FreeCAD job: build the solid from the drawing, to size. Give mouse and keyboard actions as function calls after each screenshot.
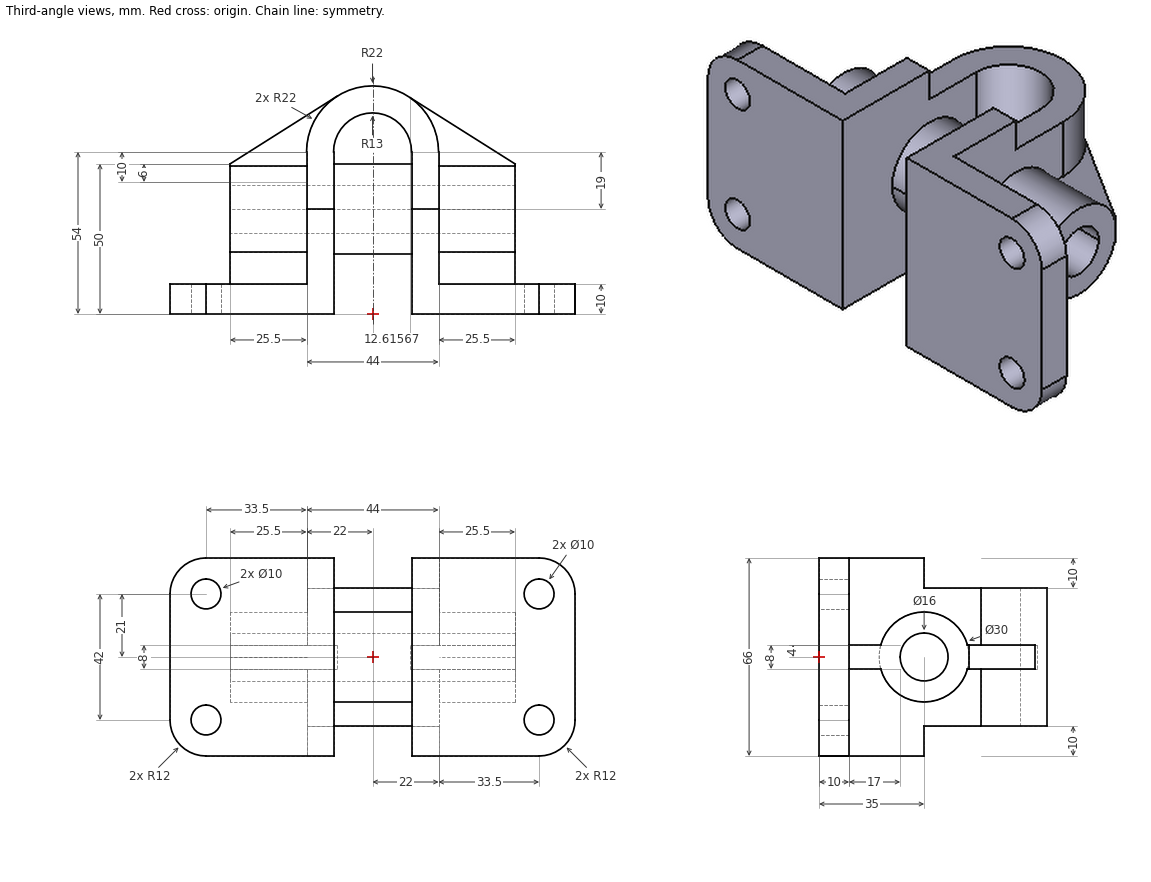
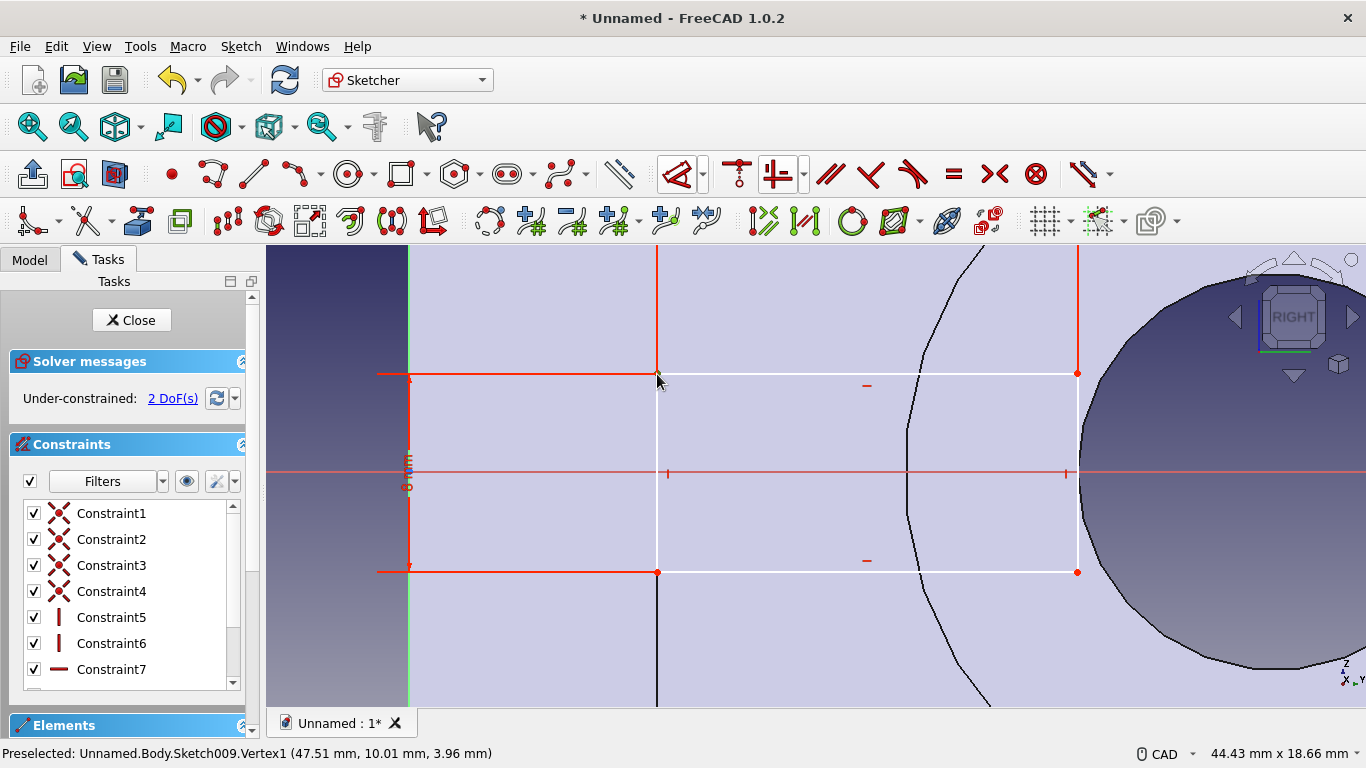
click(702, 174)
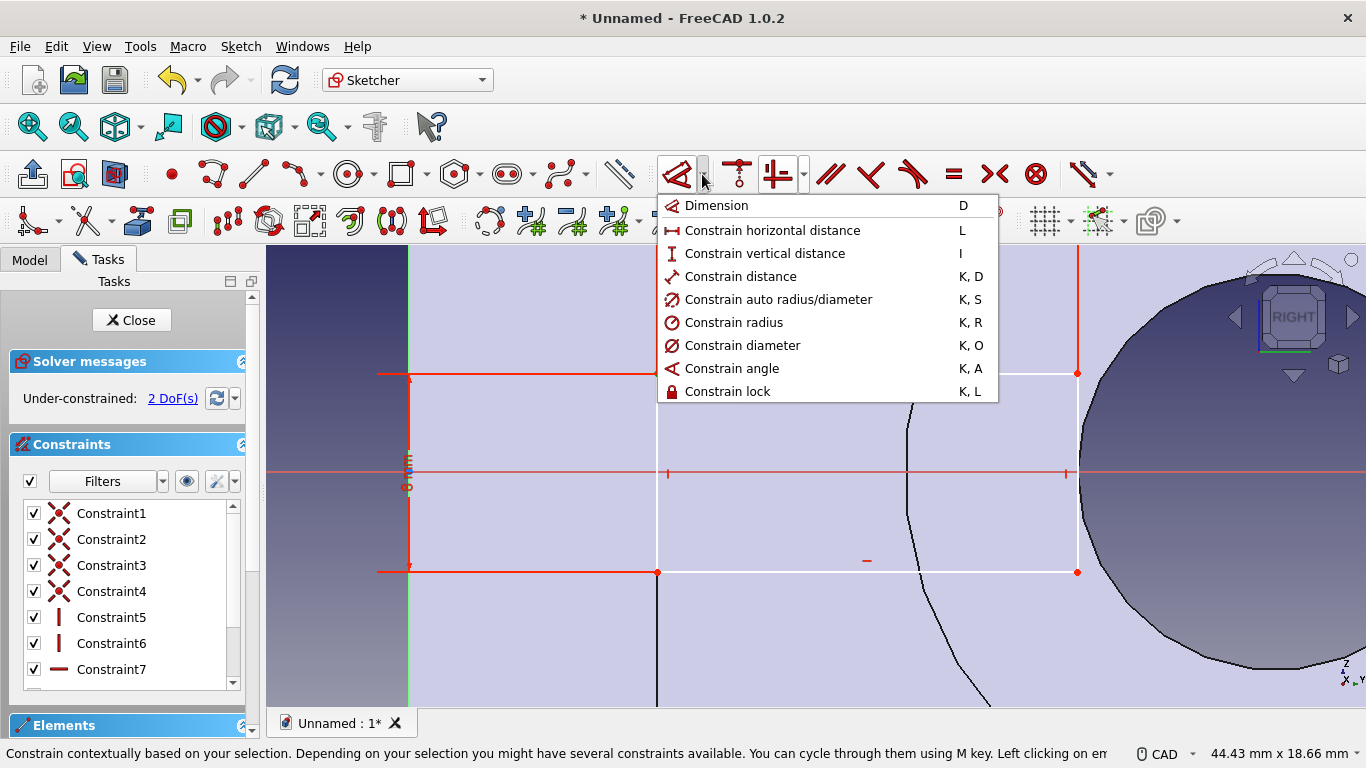
click(828, 254)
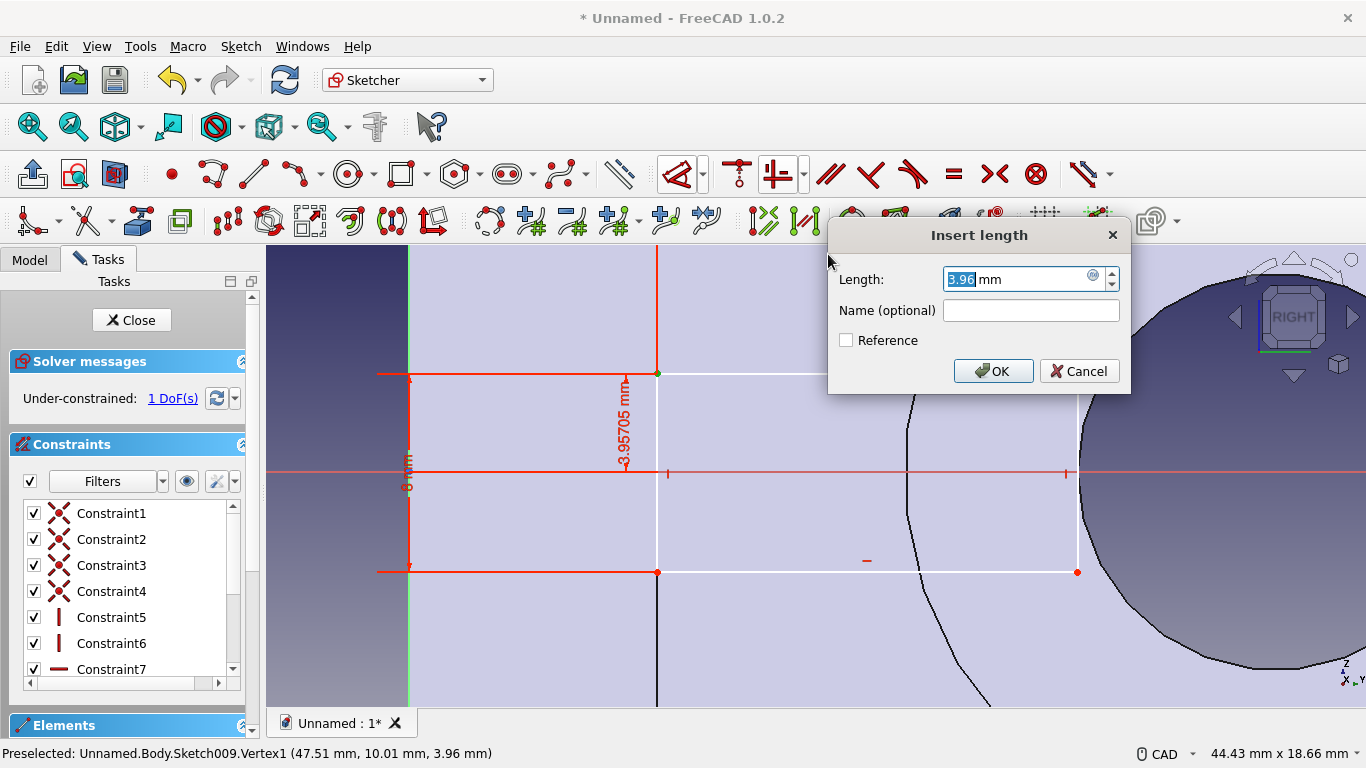
text(4)
key(Return)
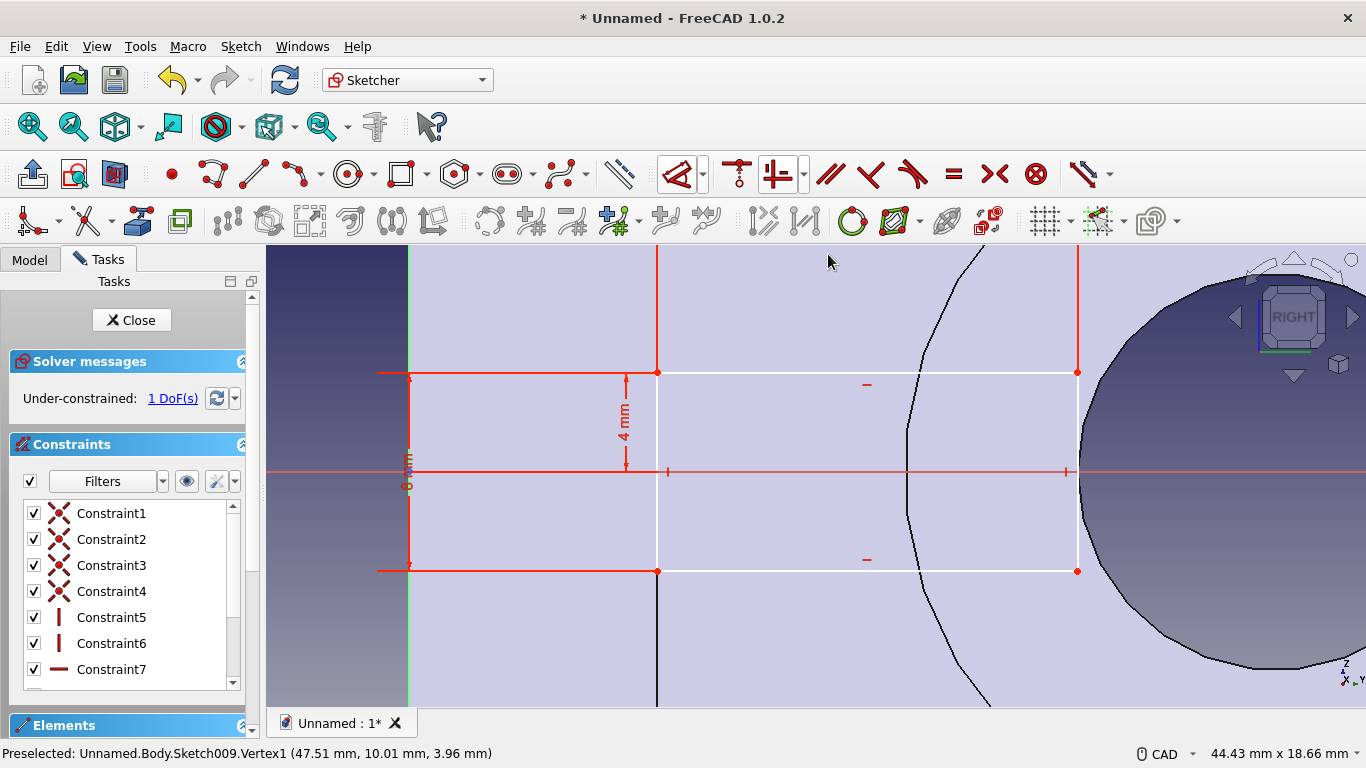
click(657, 373)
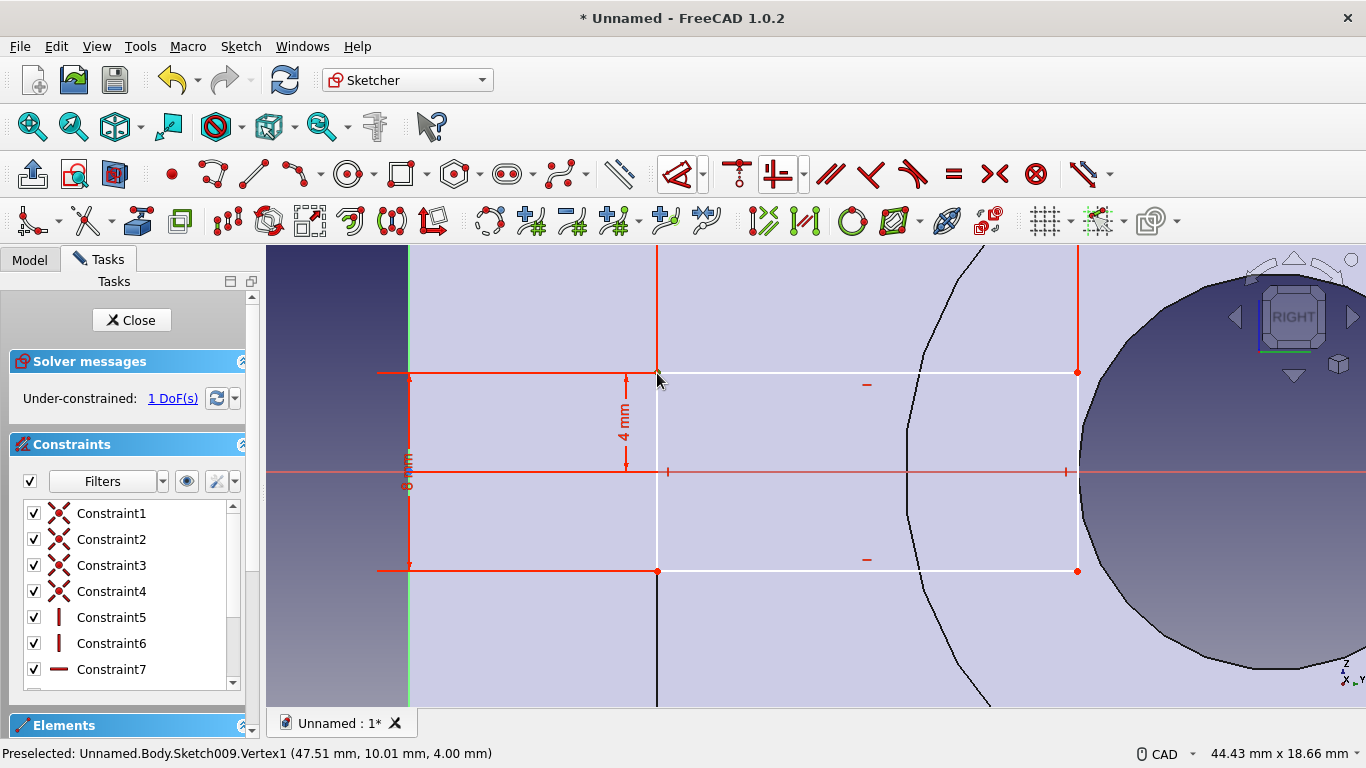
click(702, 174)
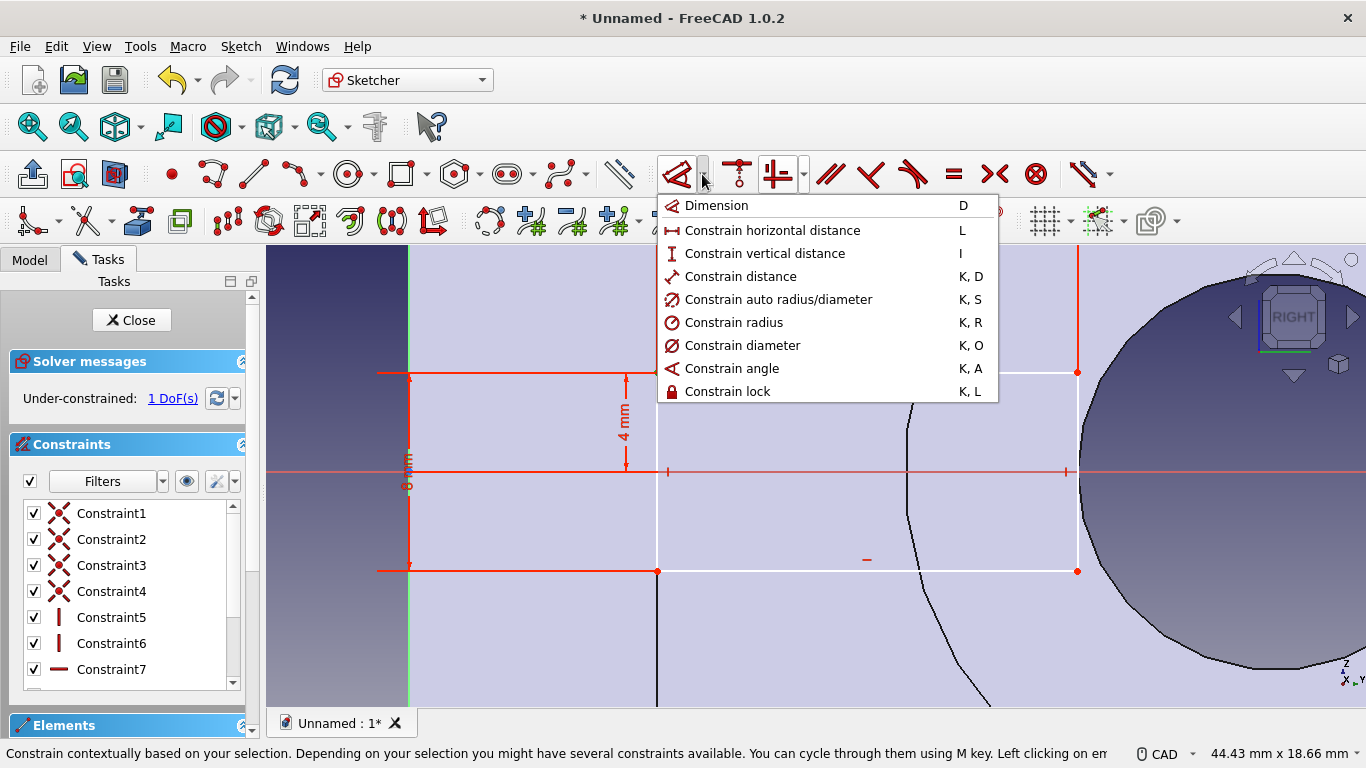
click(828, 230)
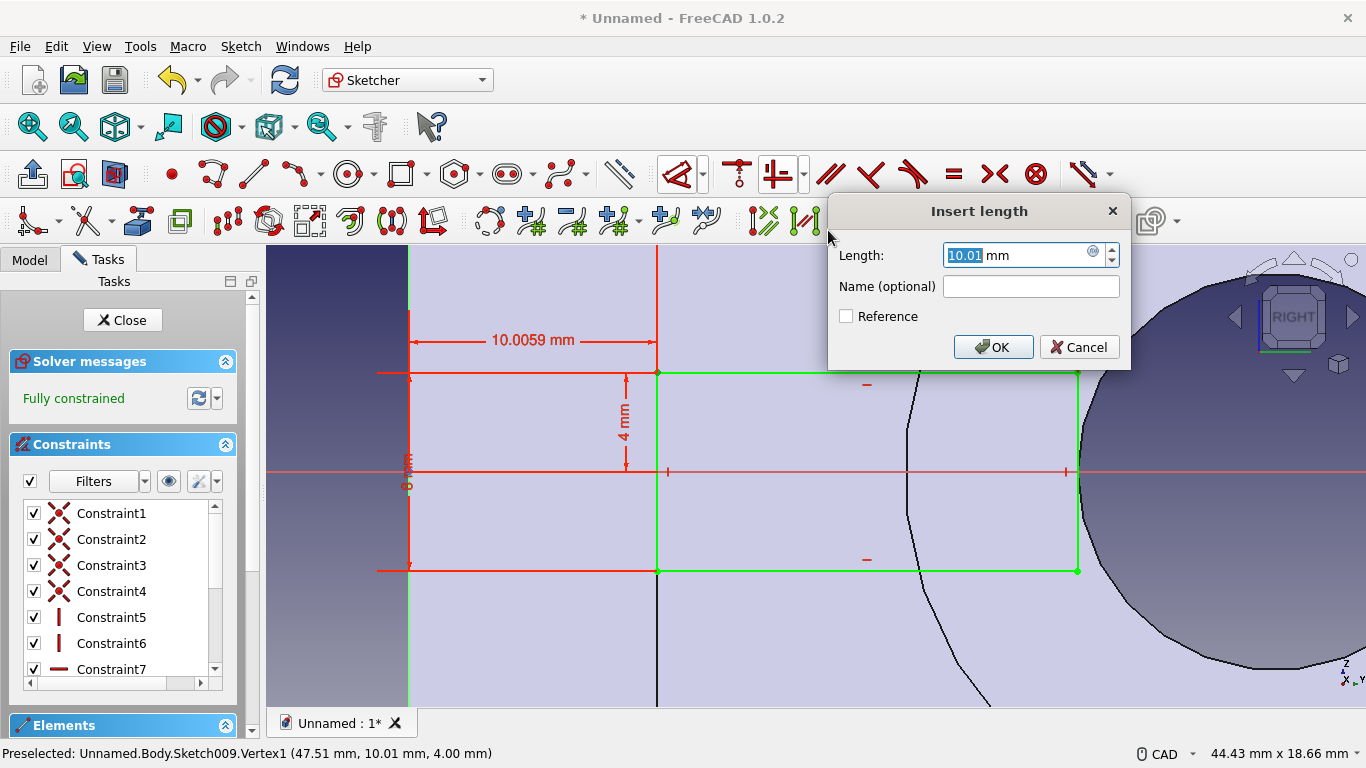
text(10)
key(Return)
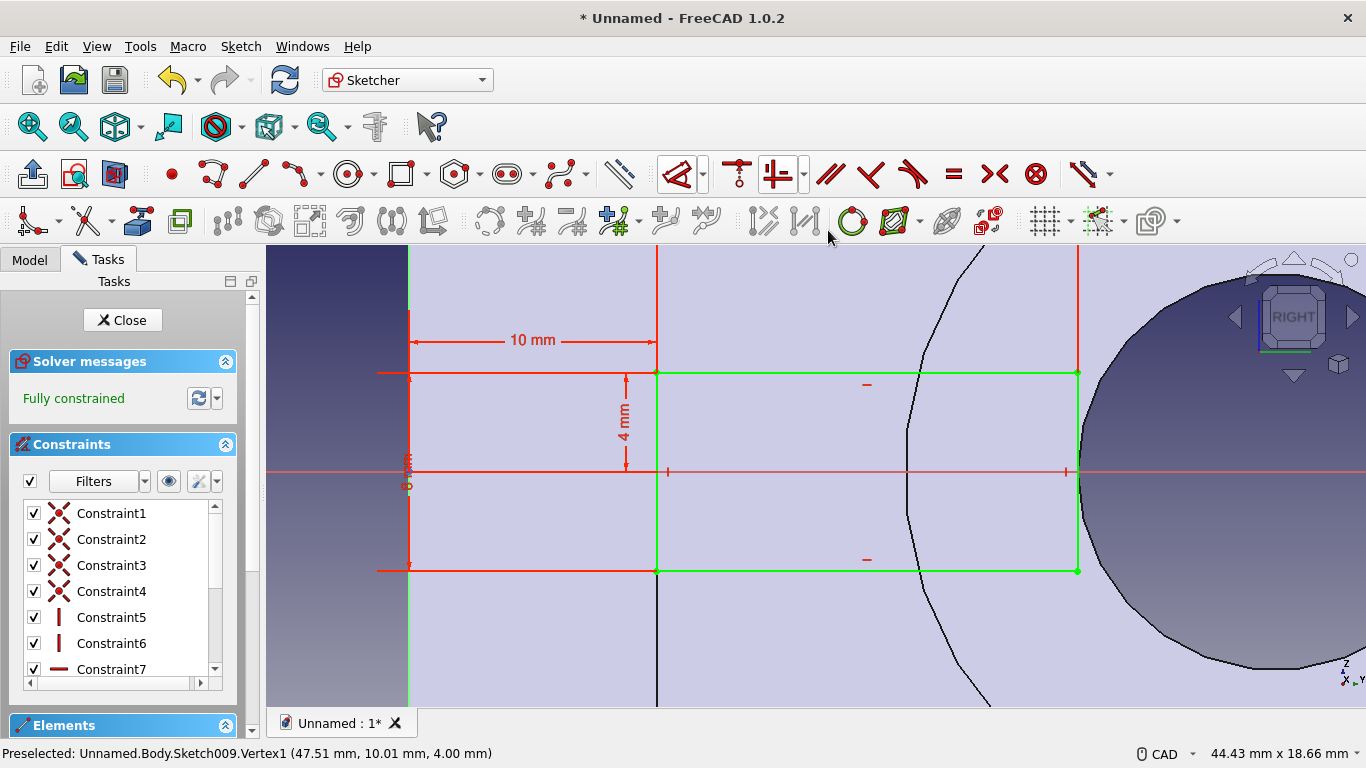
click(123, 320)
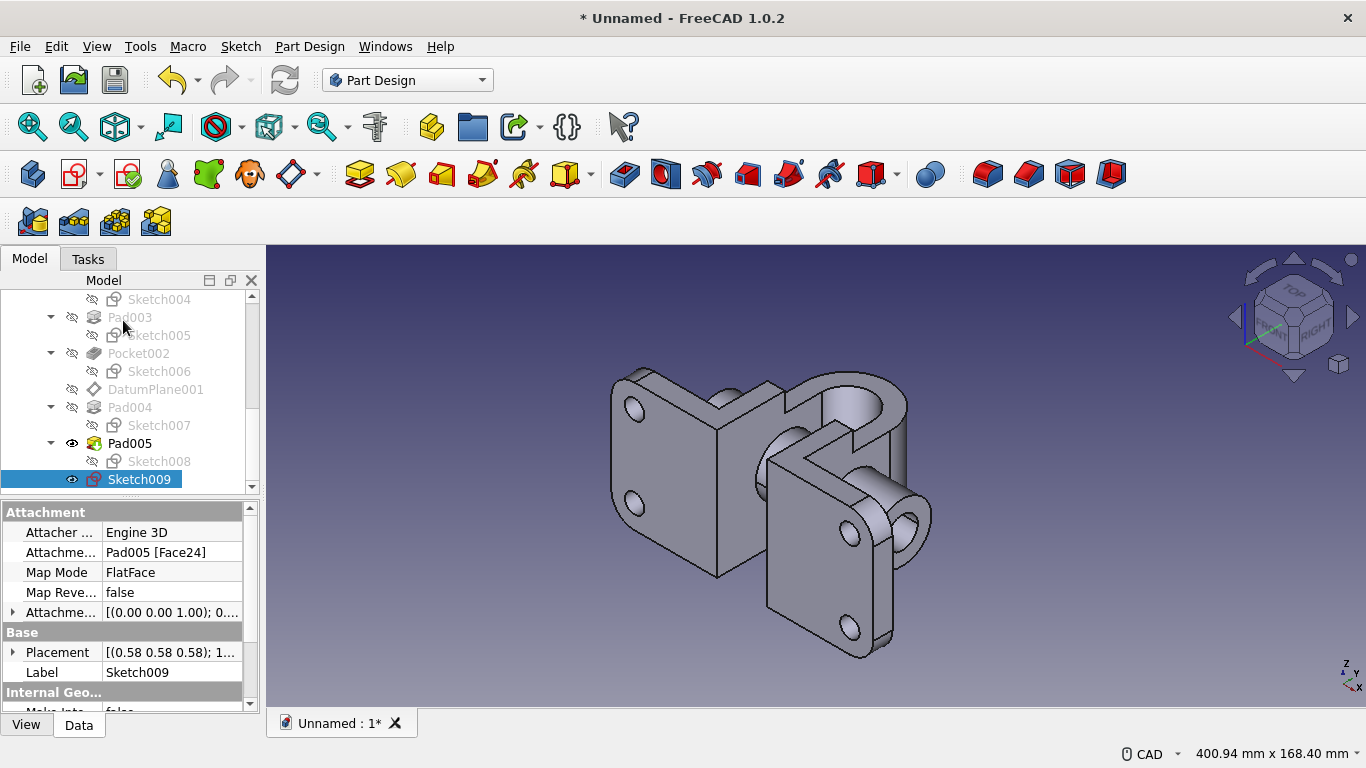
click(360, 174)